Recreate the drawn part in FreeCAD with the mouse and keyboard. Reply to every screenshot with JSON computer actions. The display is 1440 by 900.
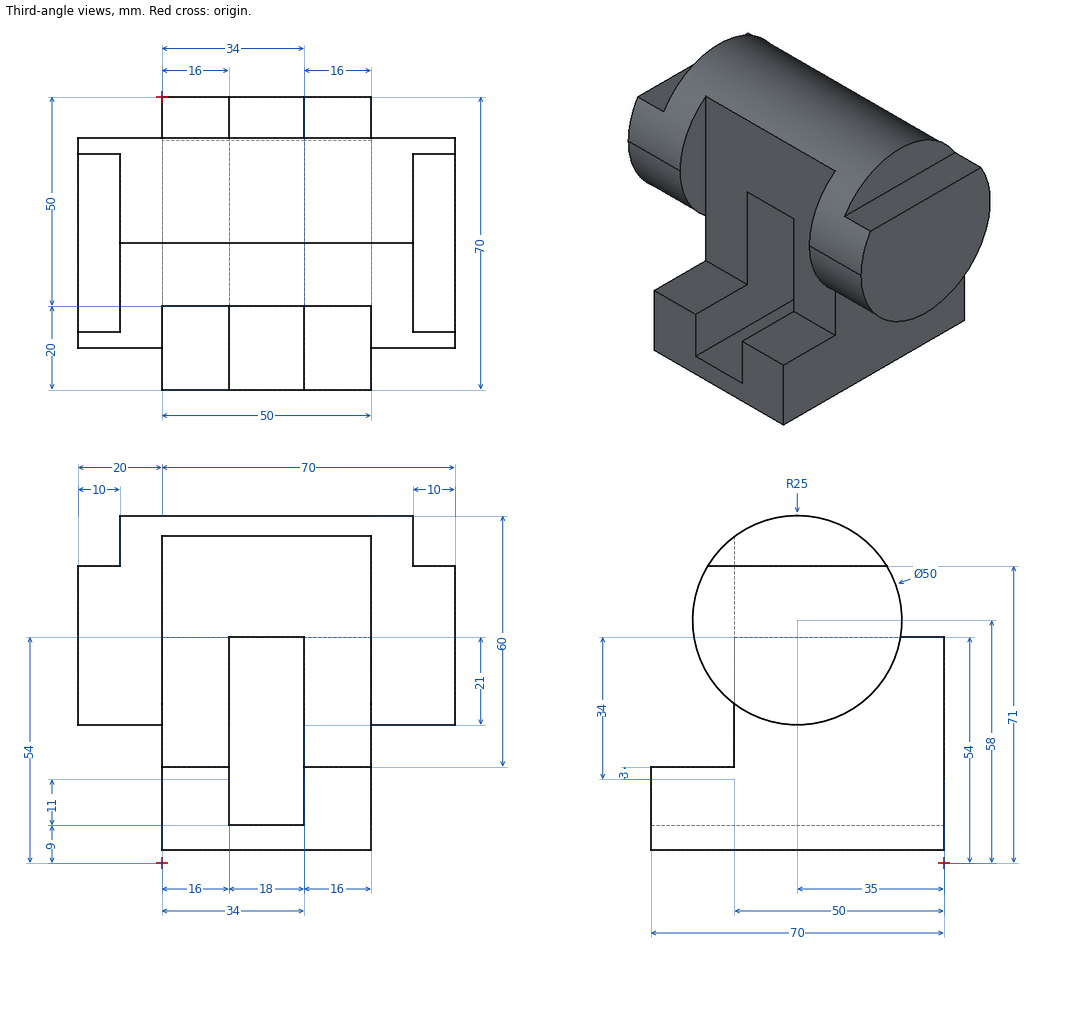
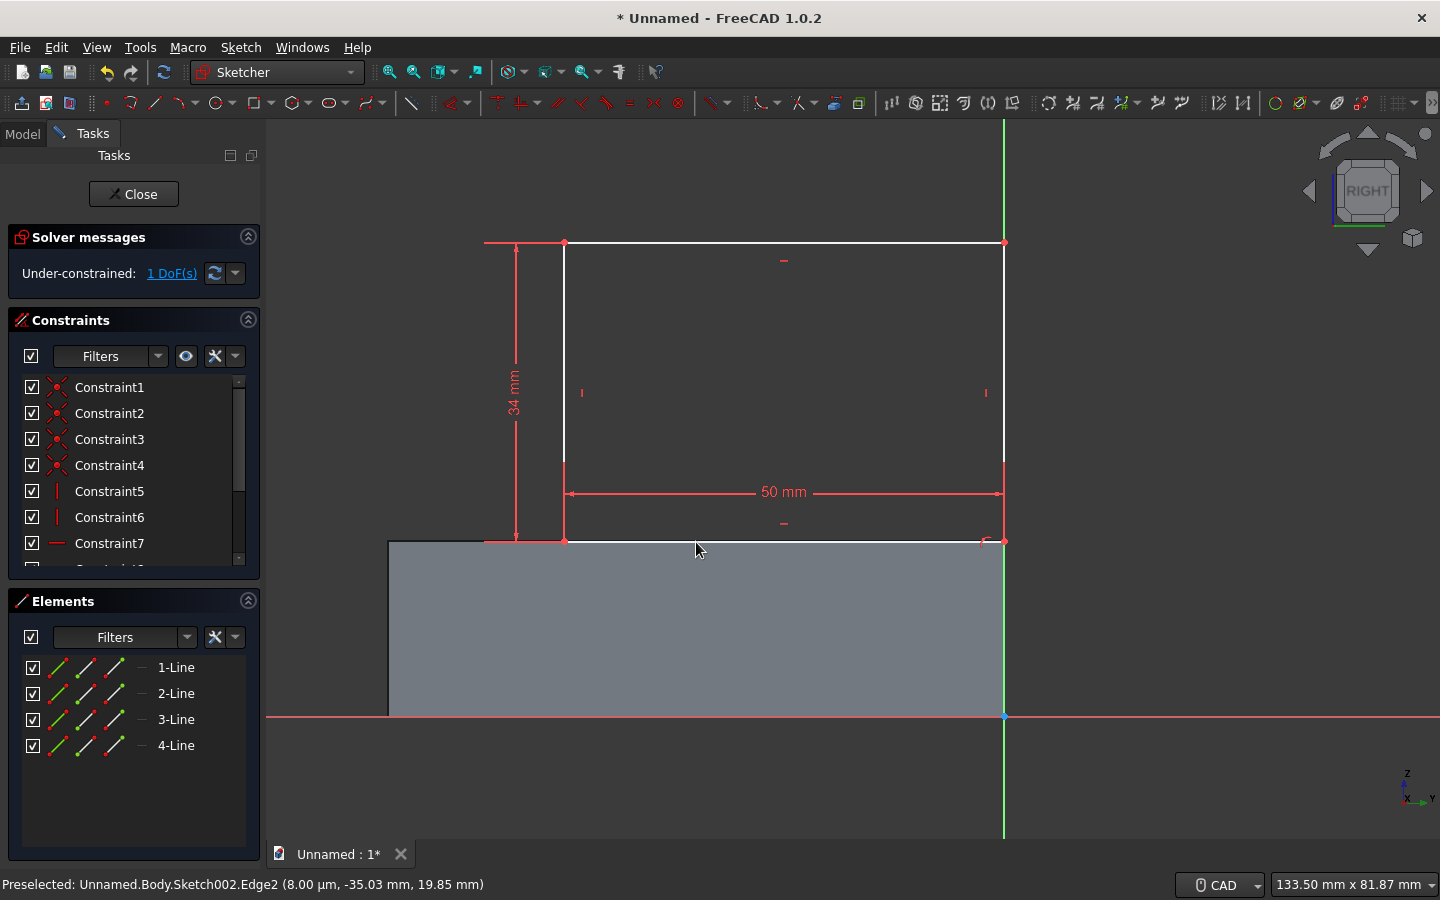
{"action": "left_click", "coordinate": [564, 243]}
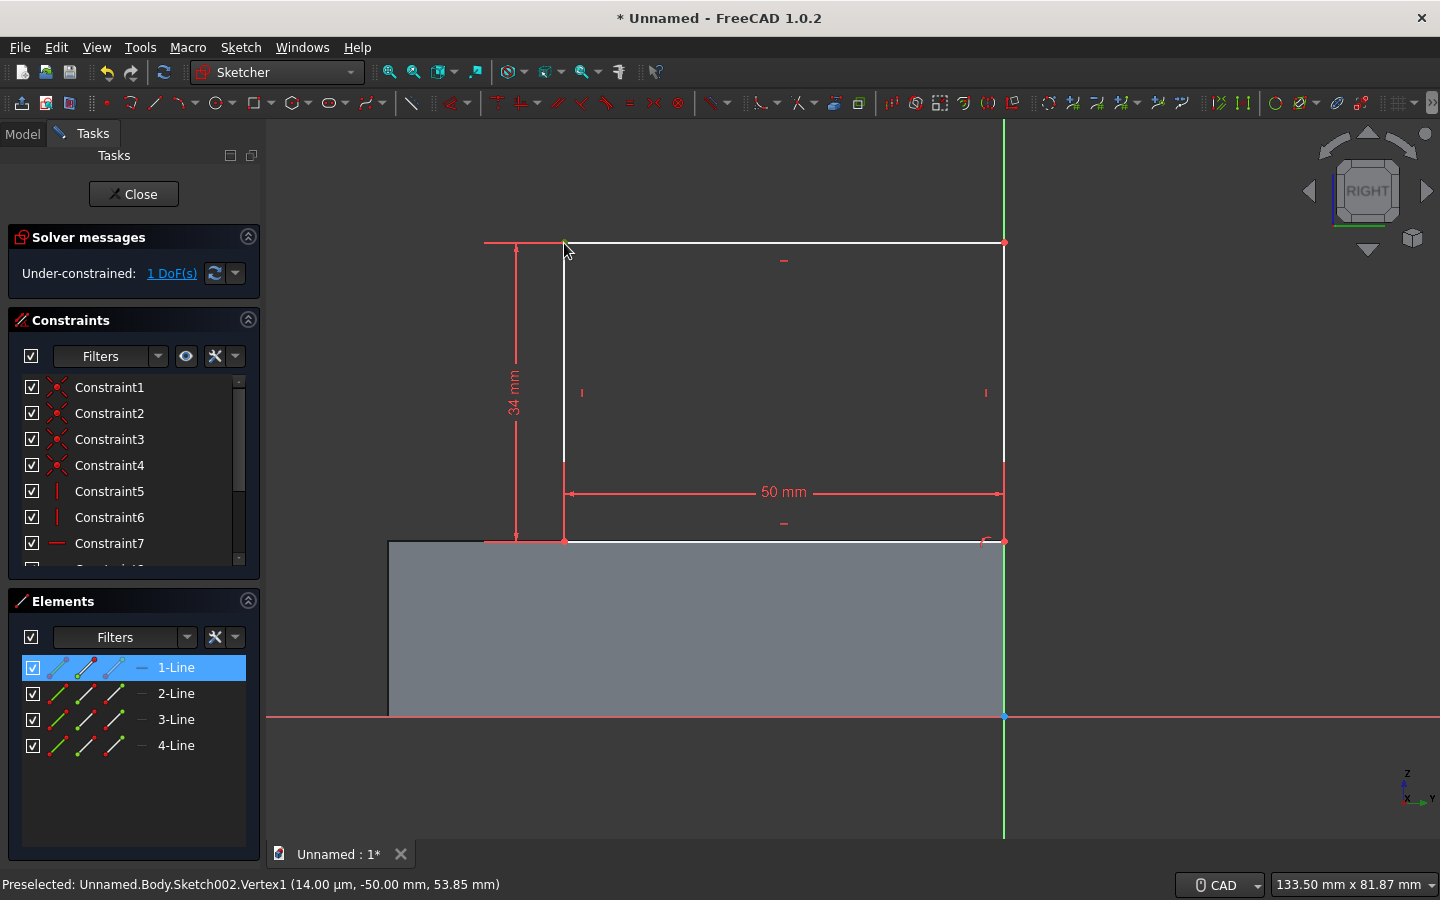
{"action": "key", "text": "i"}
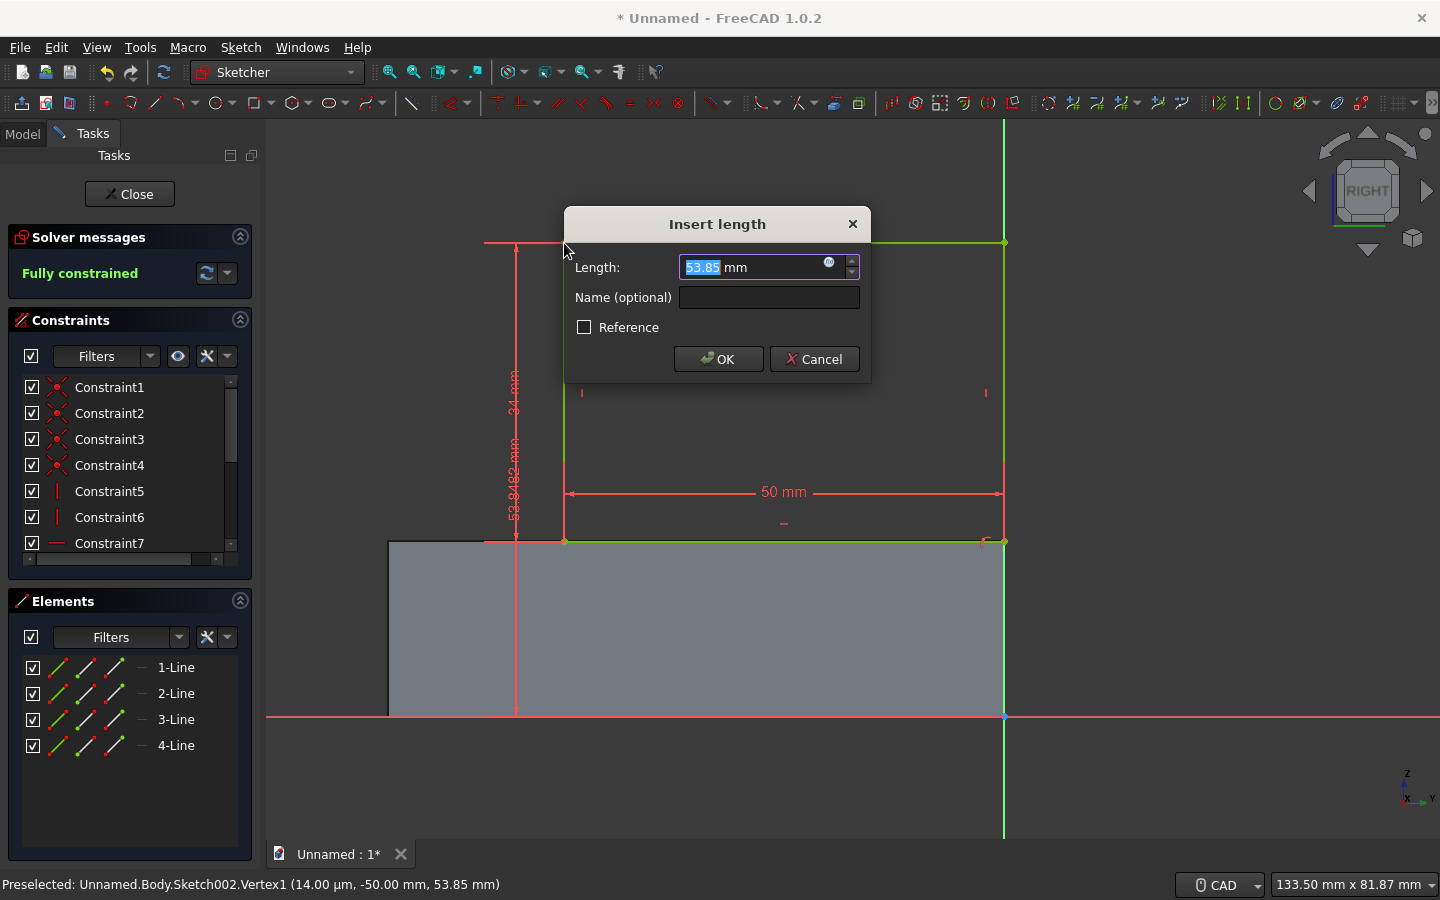
{"action": "type", "text": "54"}
{"action": "key", "text": "Return"}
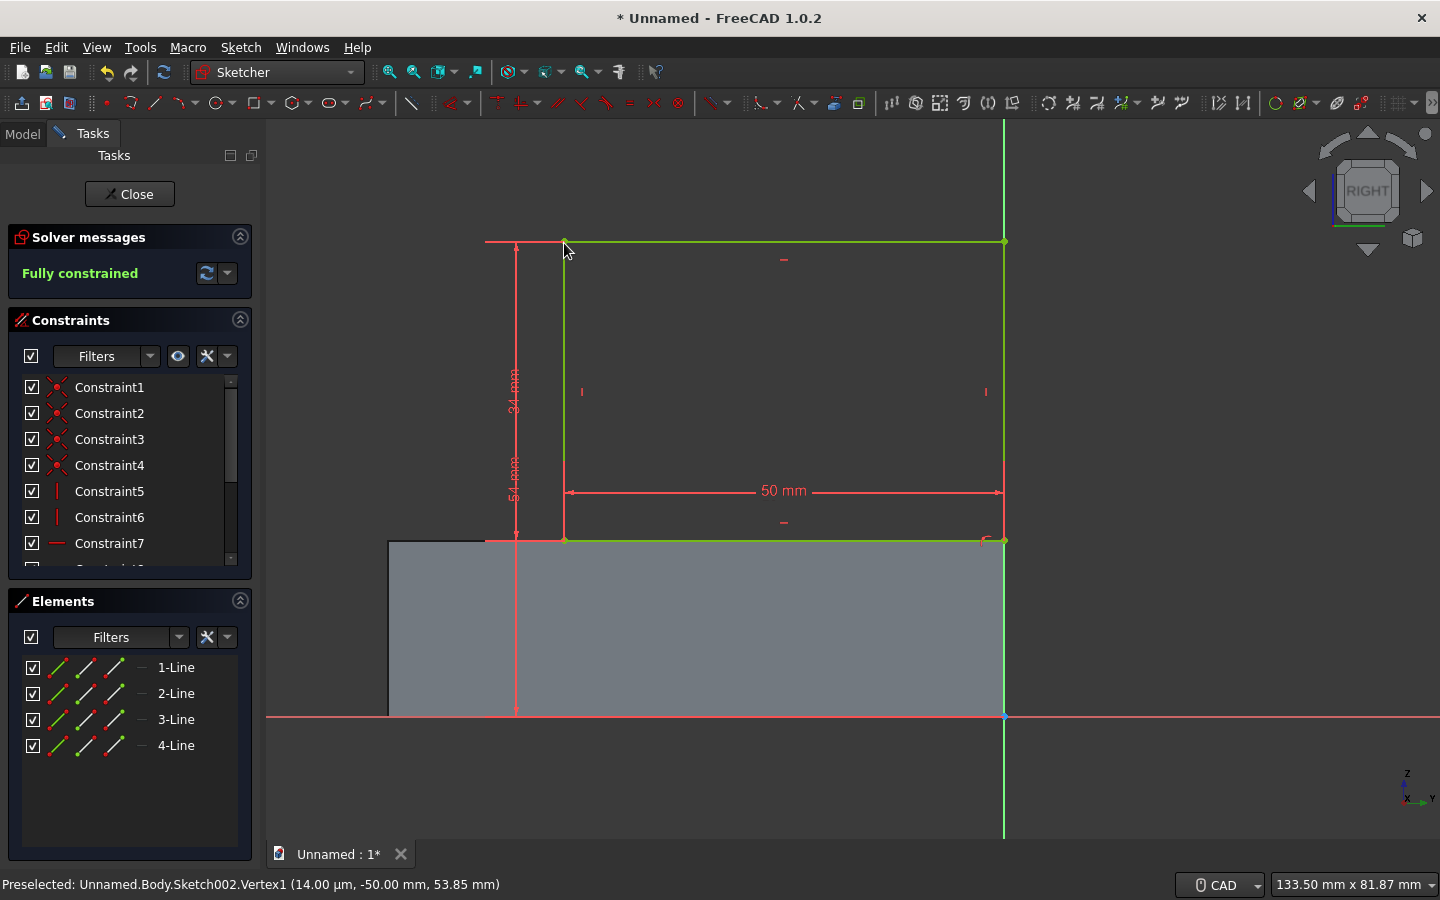
{"action": "left_click", "coordinate": [130, 194]}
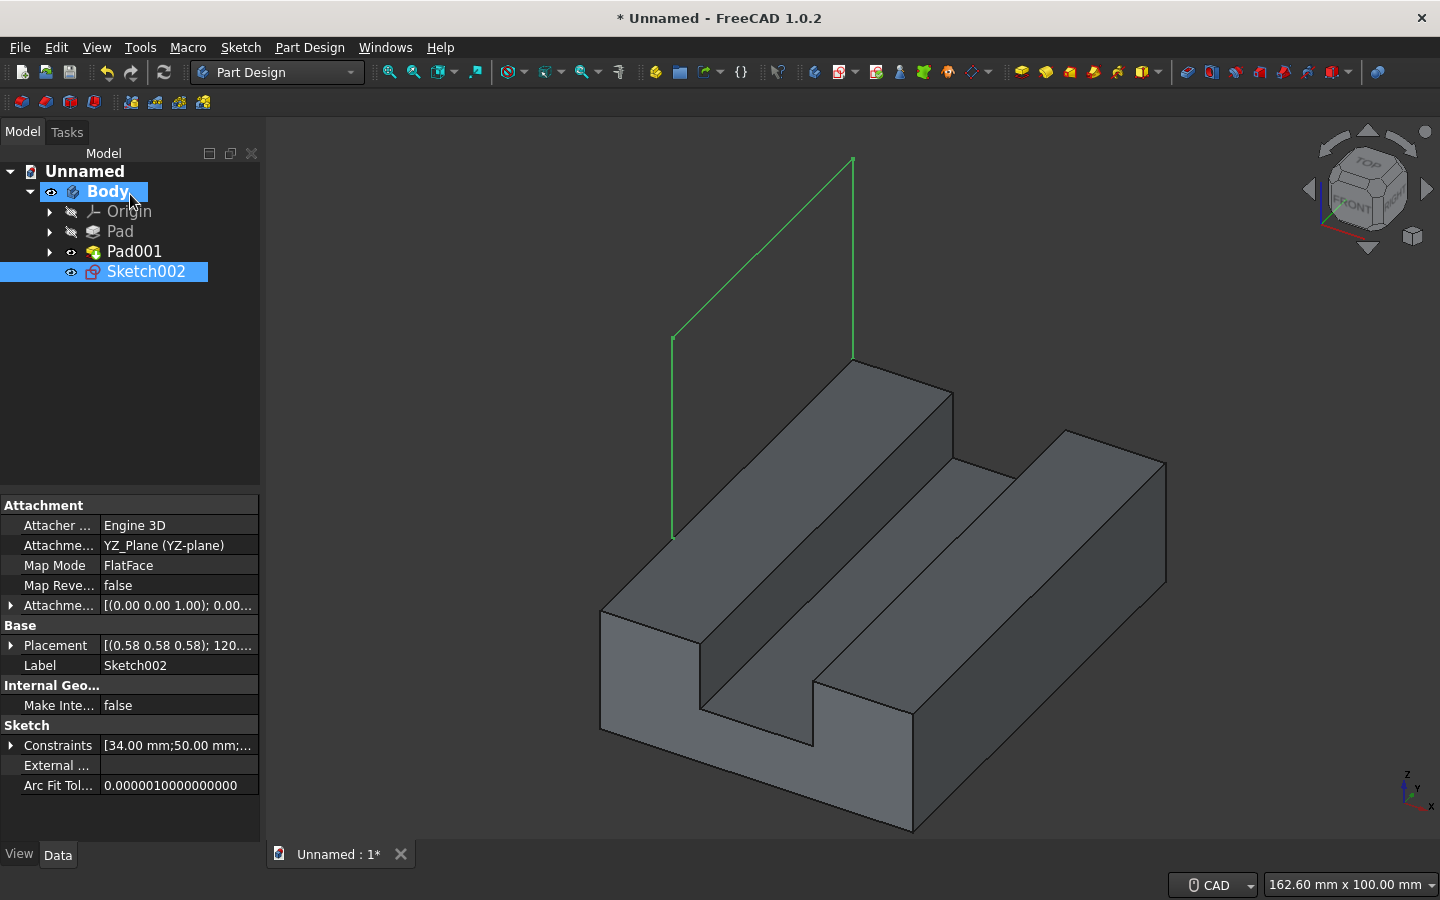
{"action": "left_click", "coordinate": [1022, 72]}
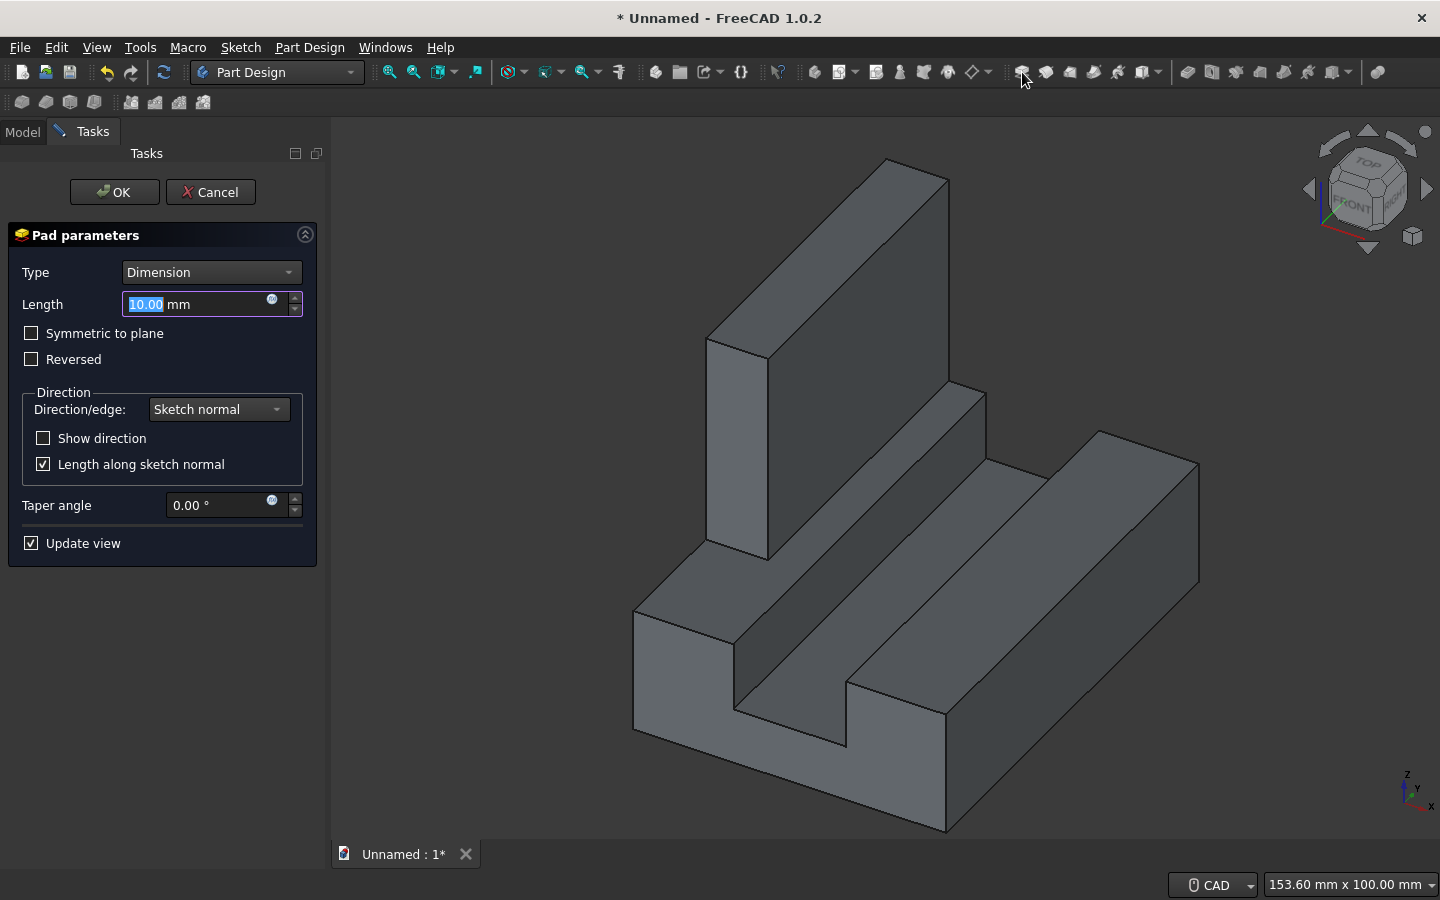
{"action": "type", "text": "16"}
{"action": "key", "text": "Tab"}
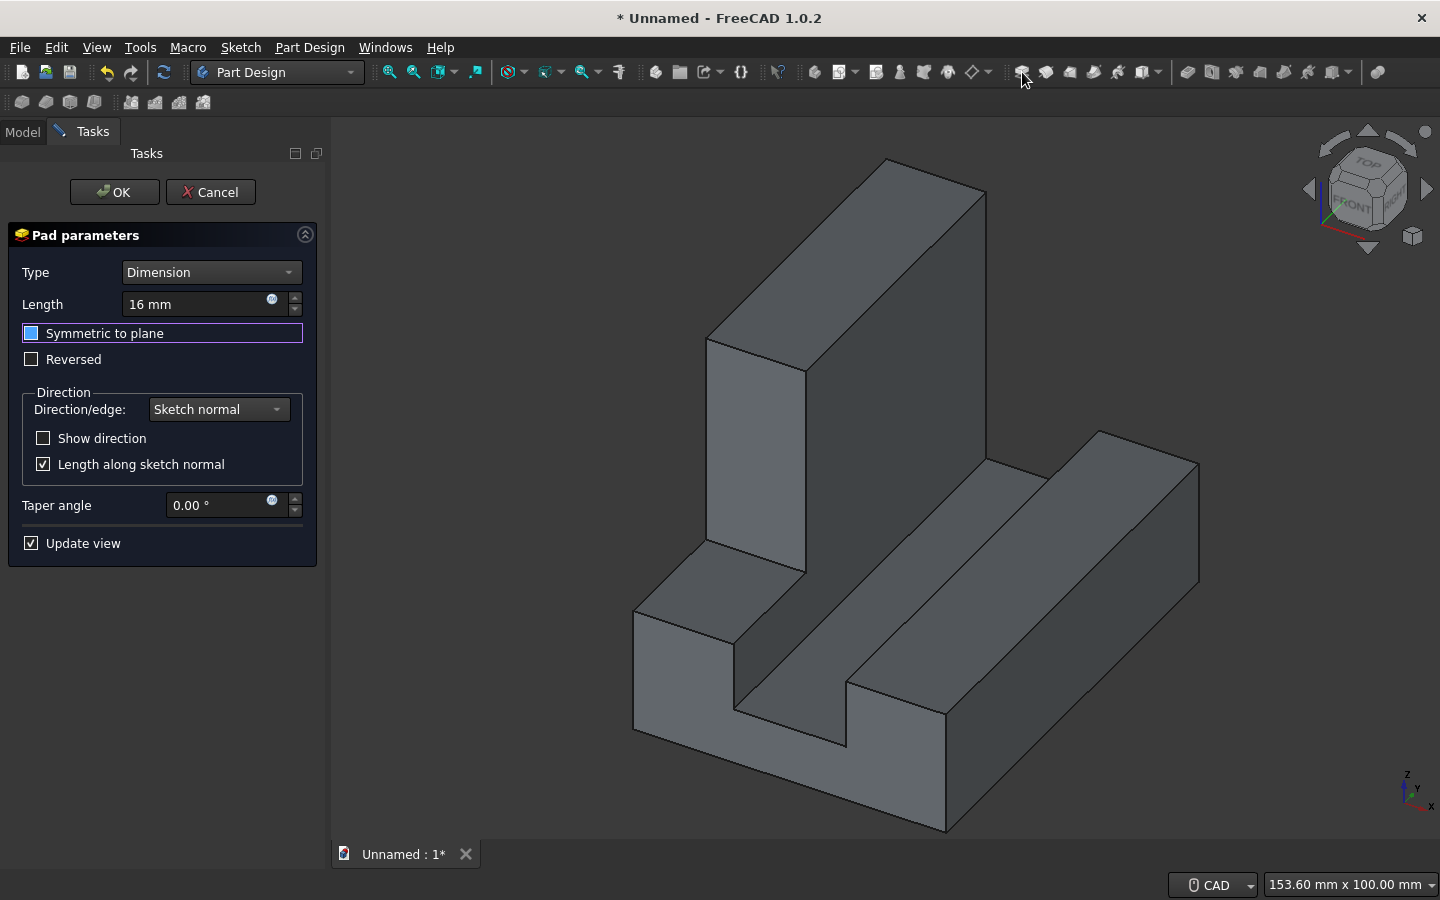
{"action": "left_click", "coordinate": [115, 192]}